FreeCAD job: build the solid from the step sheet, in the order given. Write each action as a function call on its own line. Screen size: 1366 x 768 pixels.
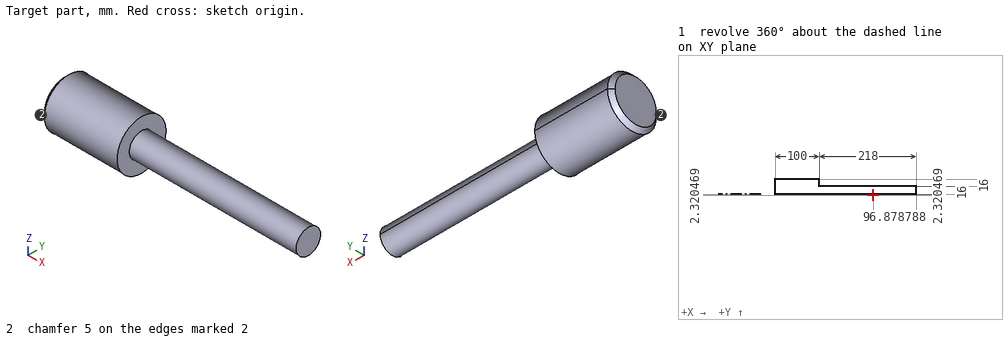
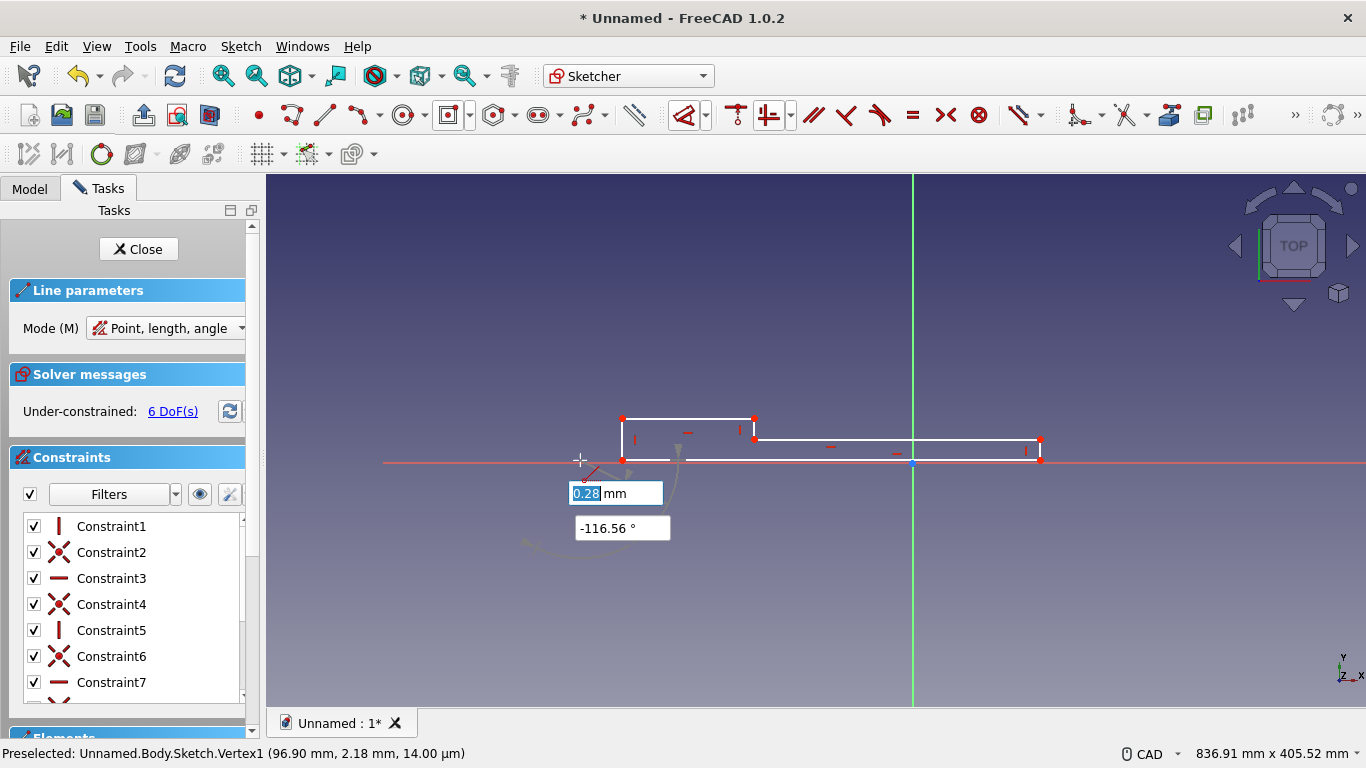
scroll(455, 460, up, 9)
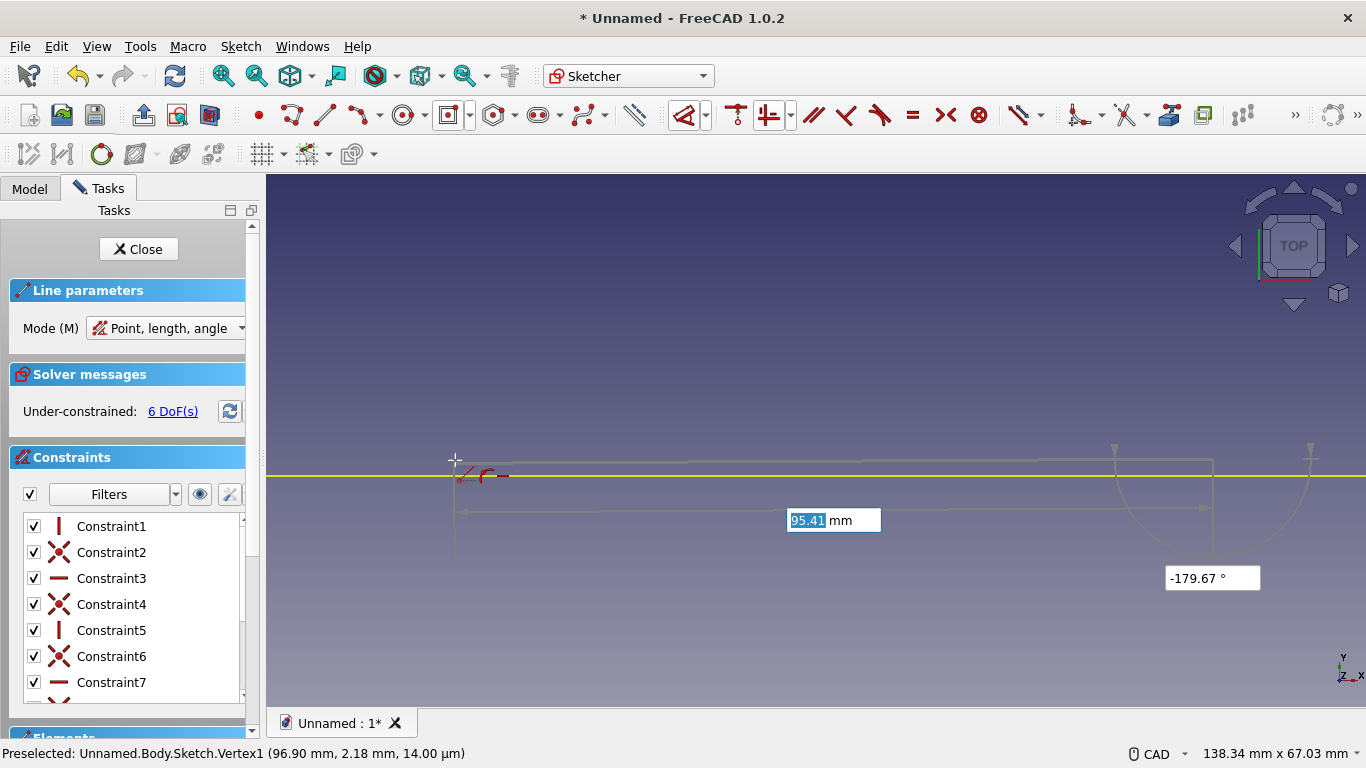
click(455, 458)
key(Escape)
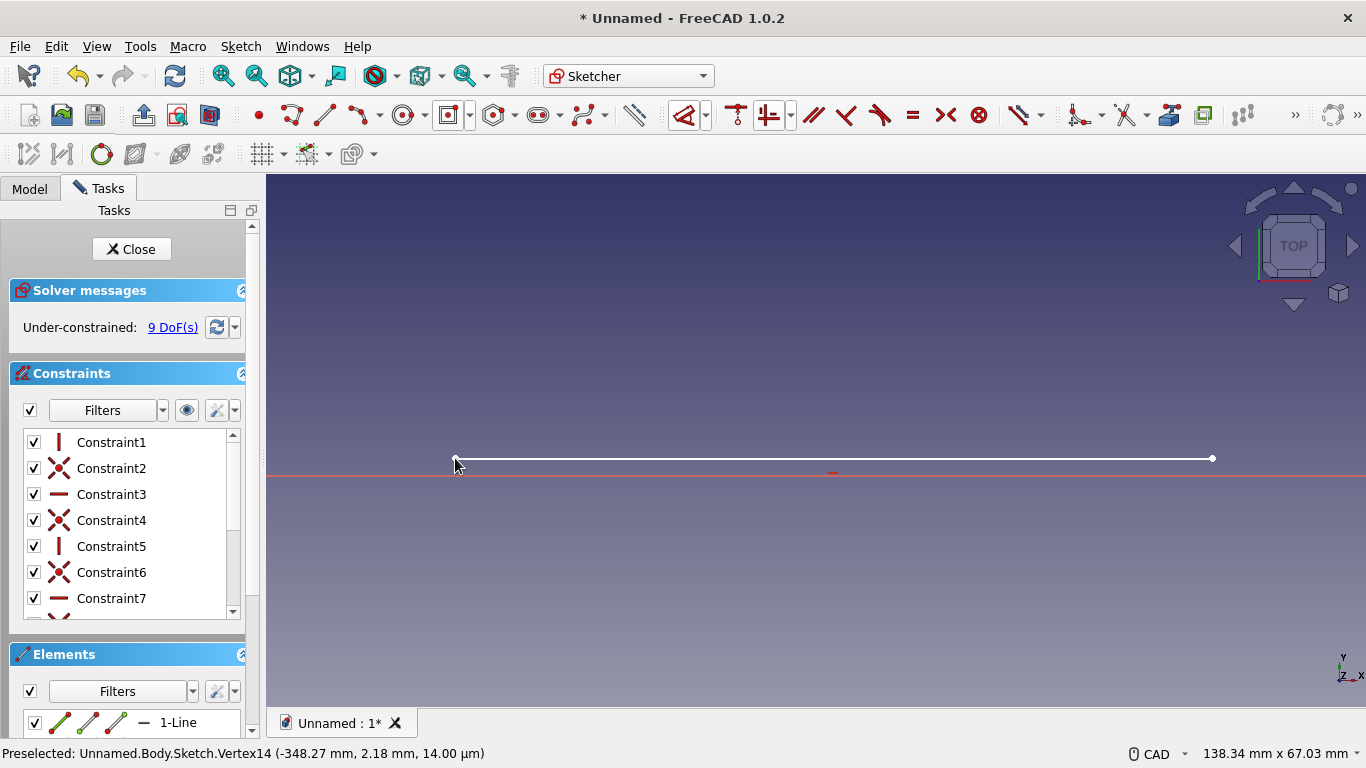
click(985, 459)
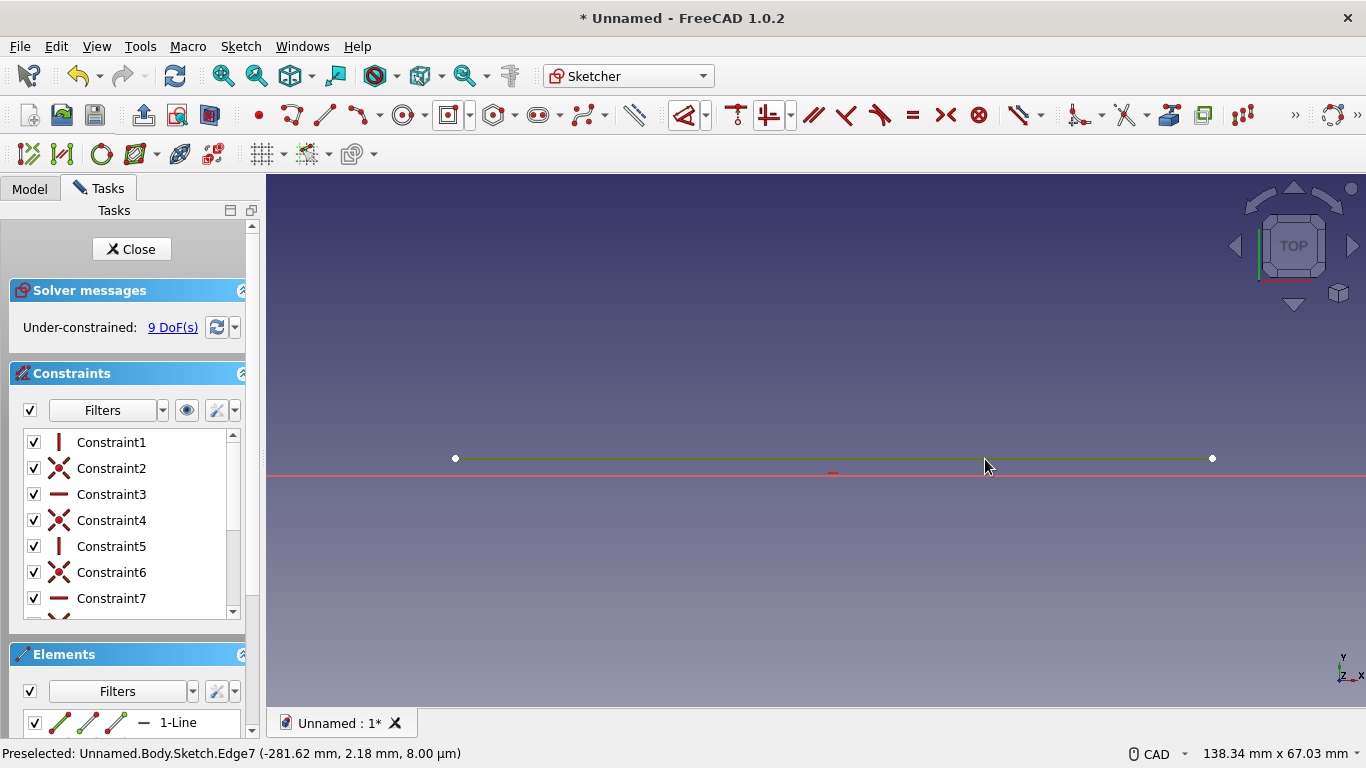
click(635, 116)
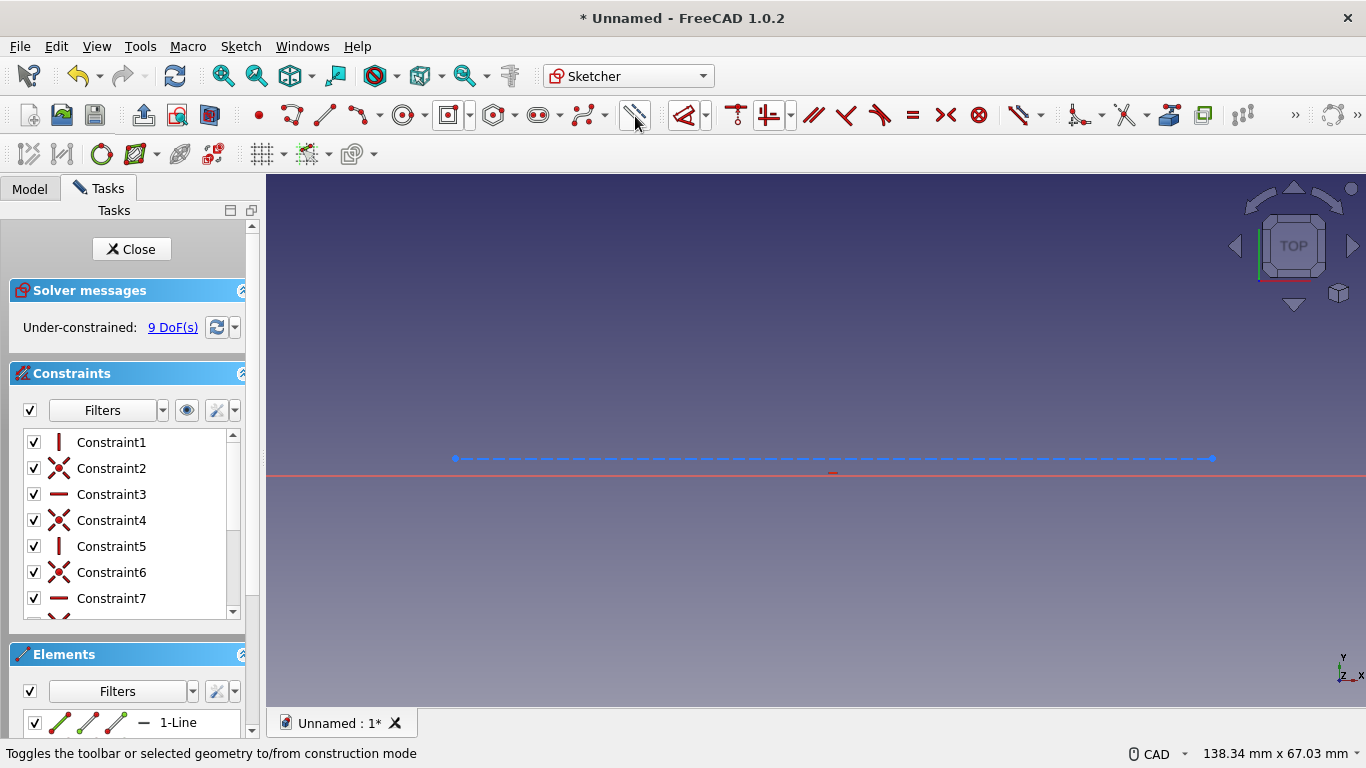
click(684, 116)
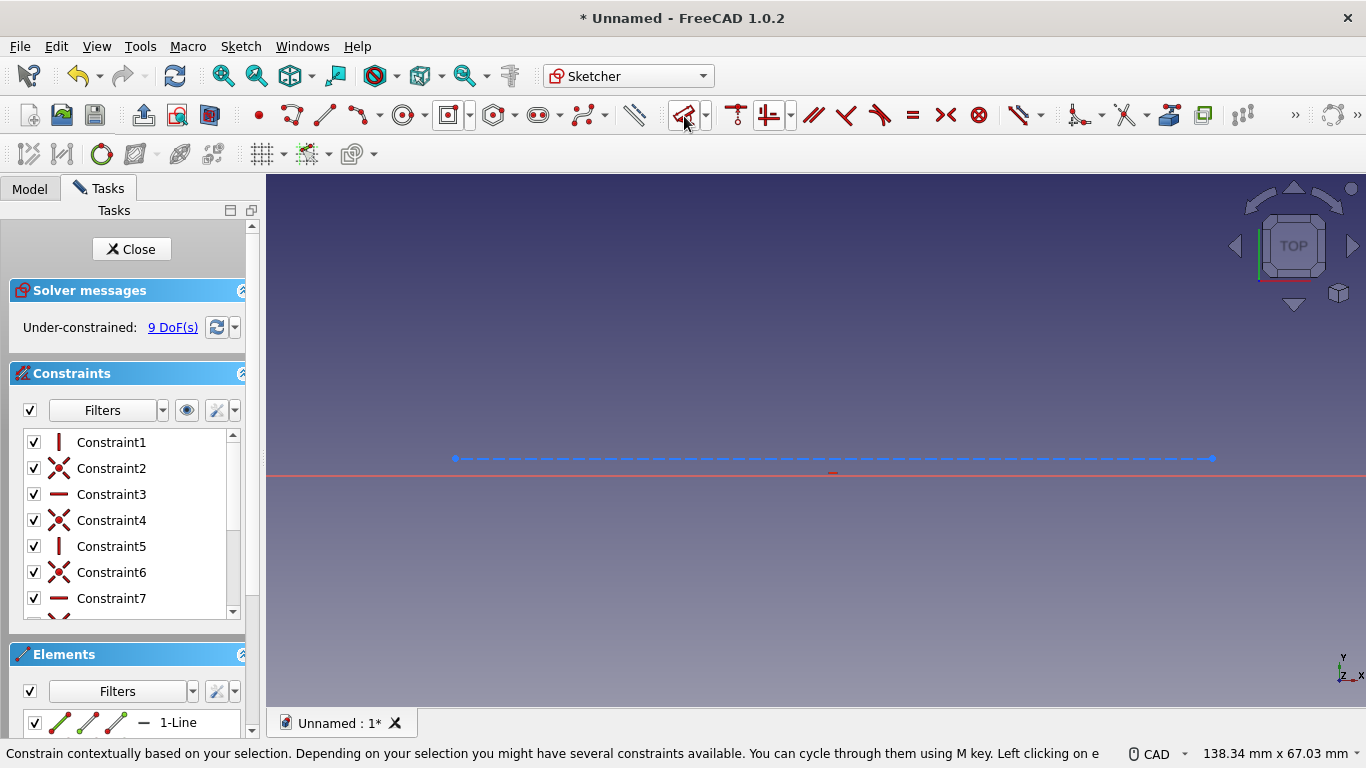
scroll(455, 460, down, 9)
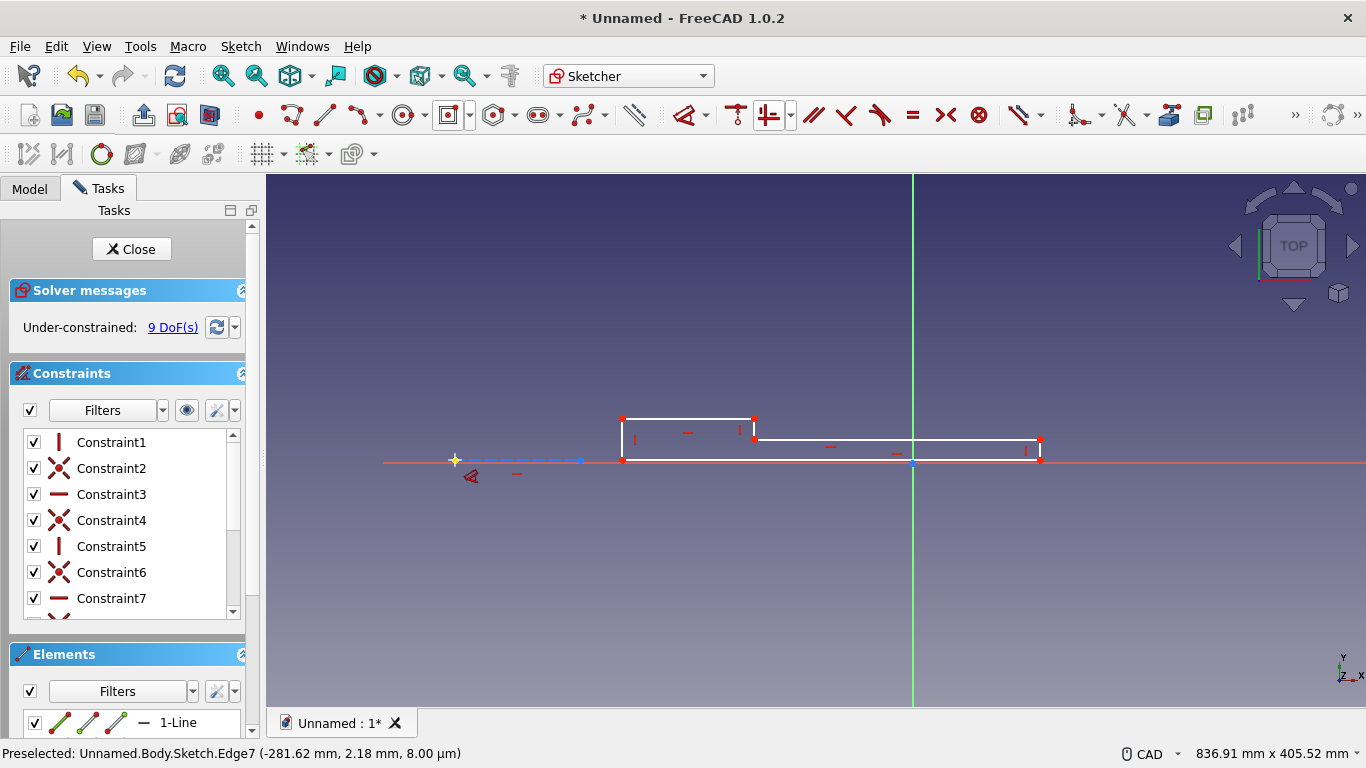
scroll(1040, 454, up, 5)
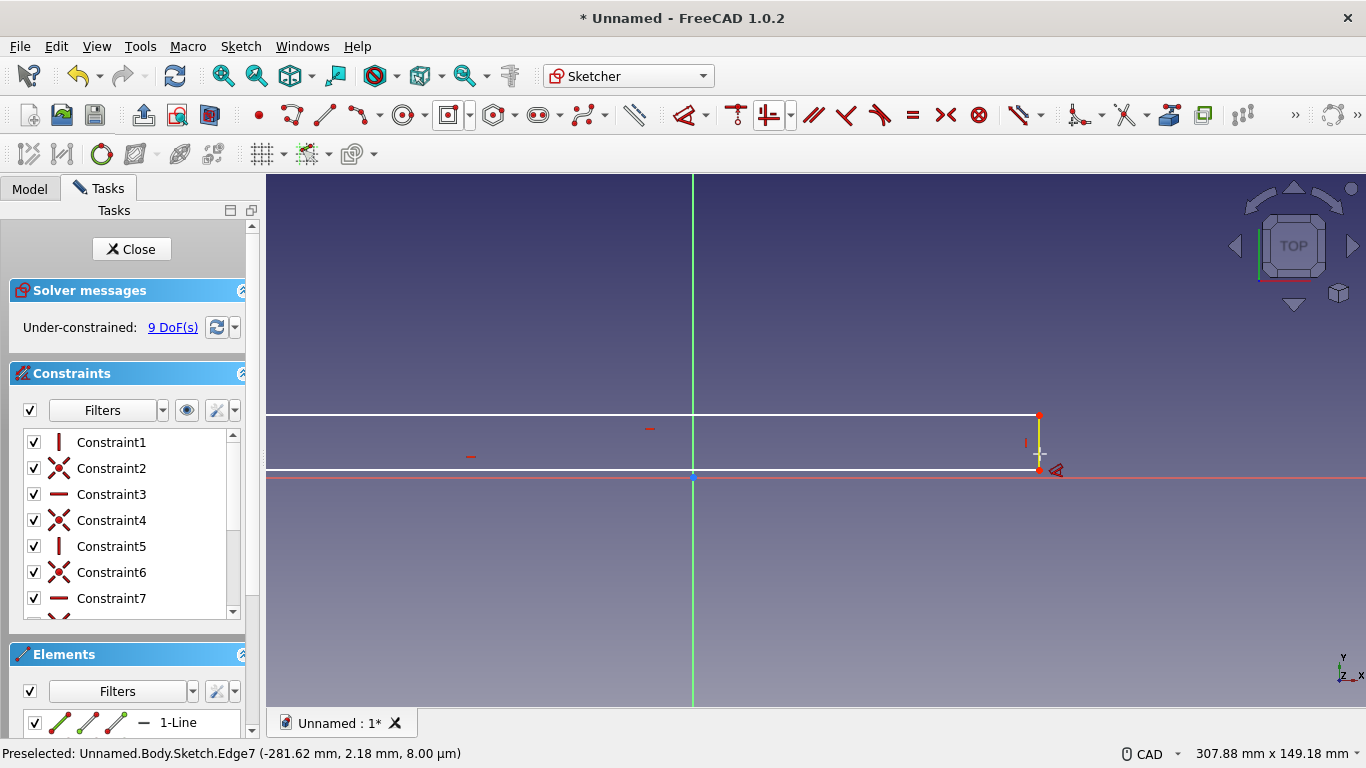
click(1039, 454)
click(1073, 443)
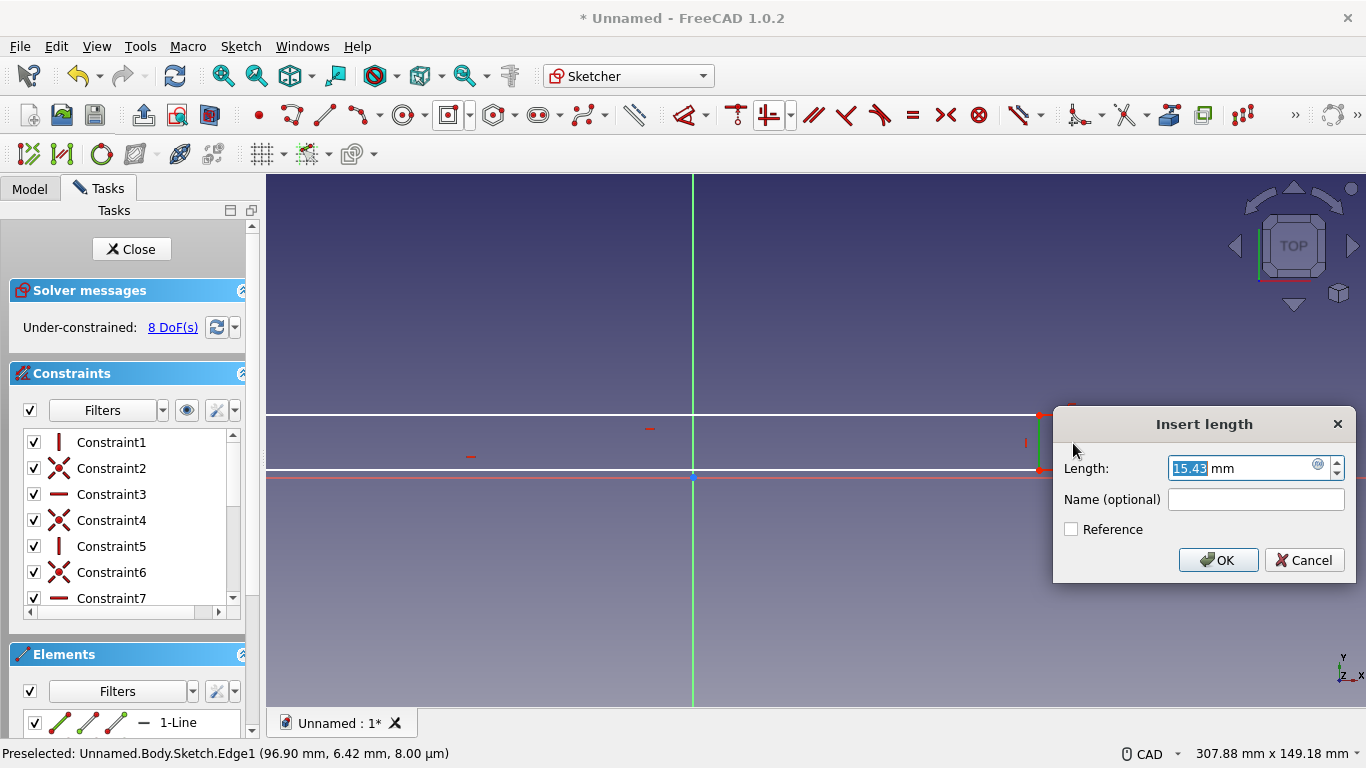
text(16)
key(Return)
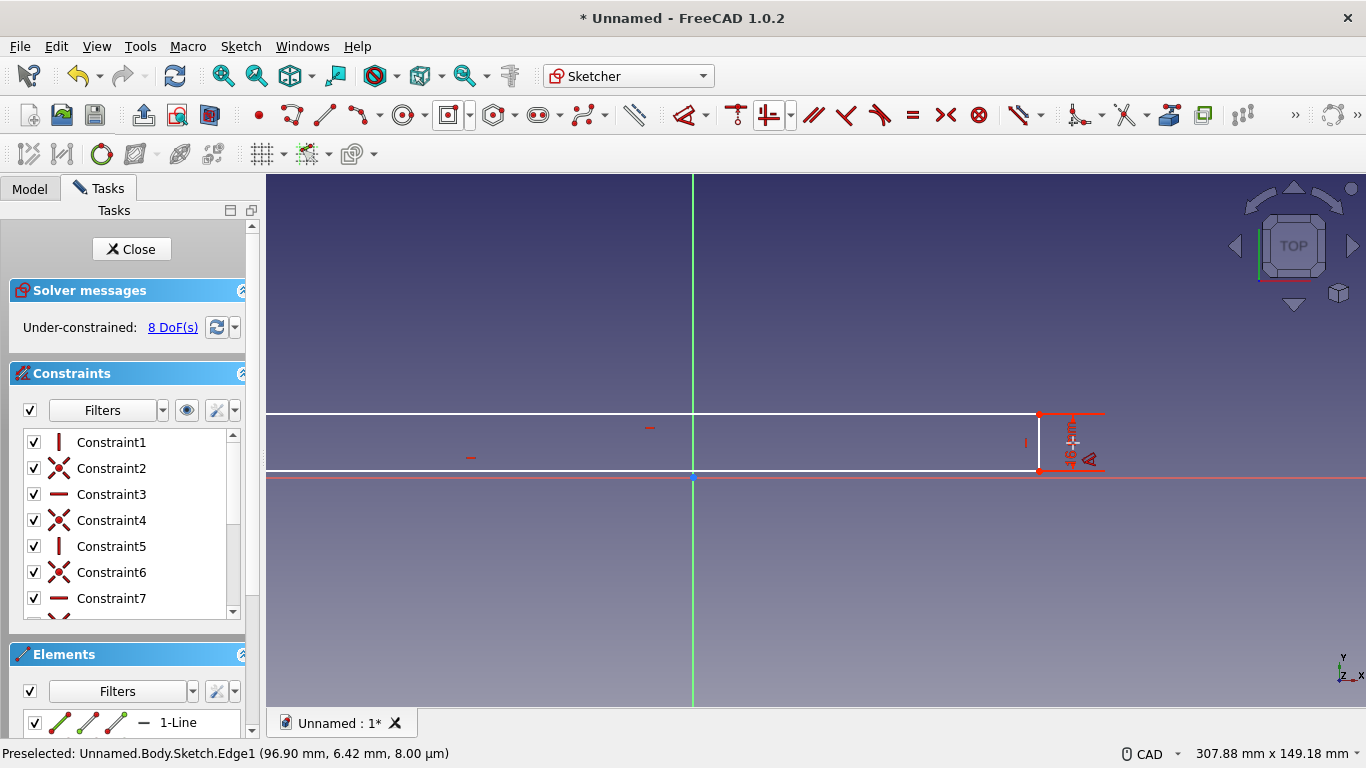
scroll(1040, 454, down, 5)